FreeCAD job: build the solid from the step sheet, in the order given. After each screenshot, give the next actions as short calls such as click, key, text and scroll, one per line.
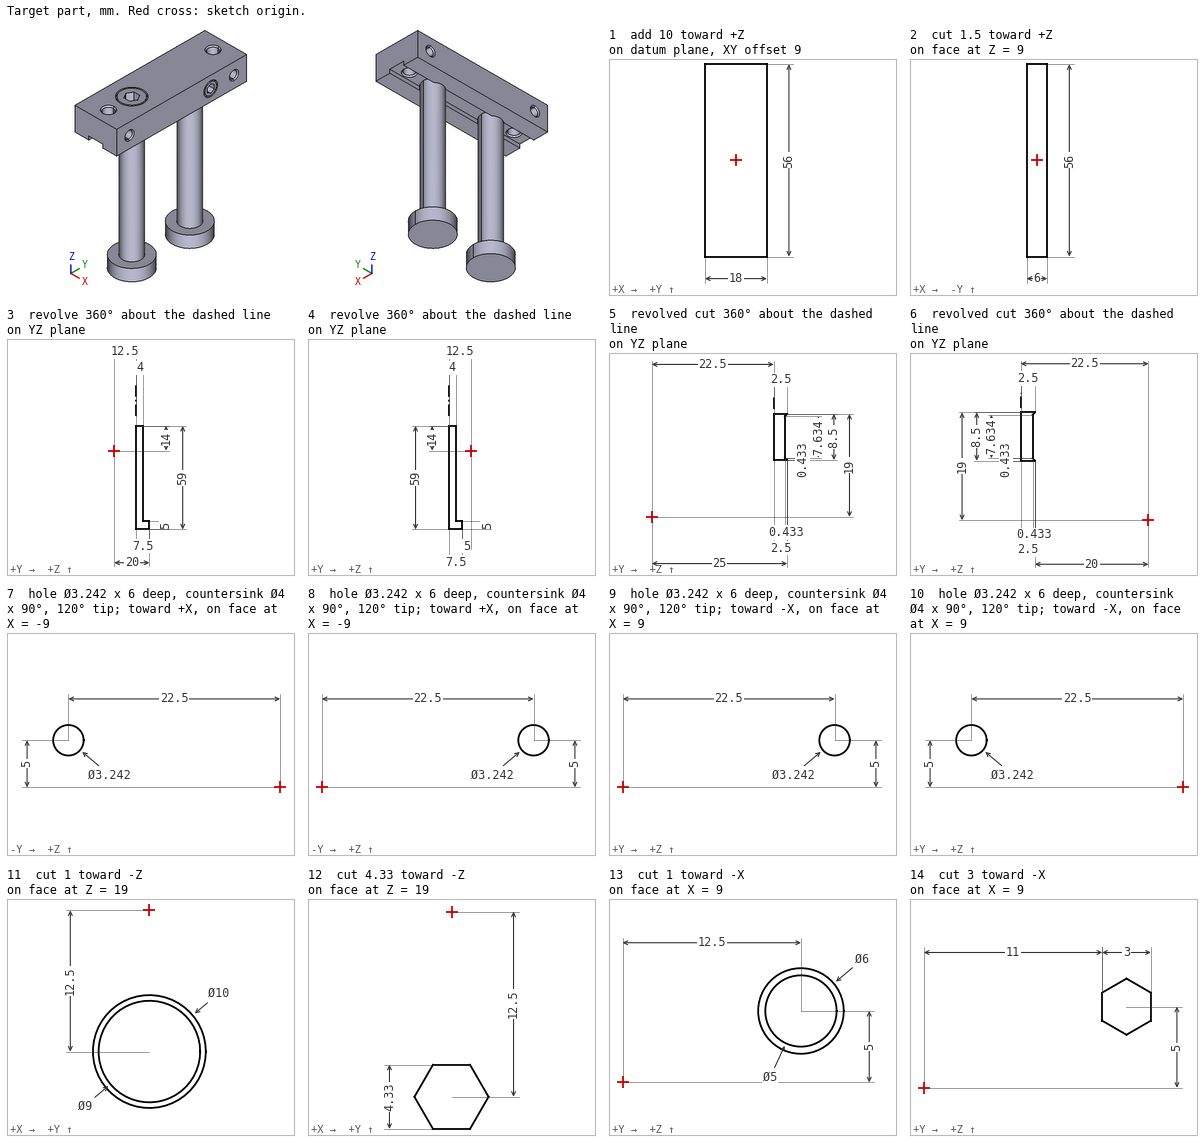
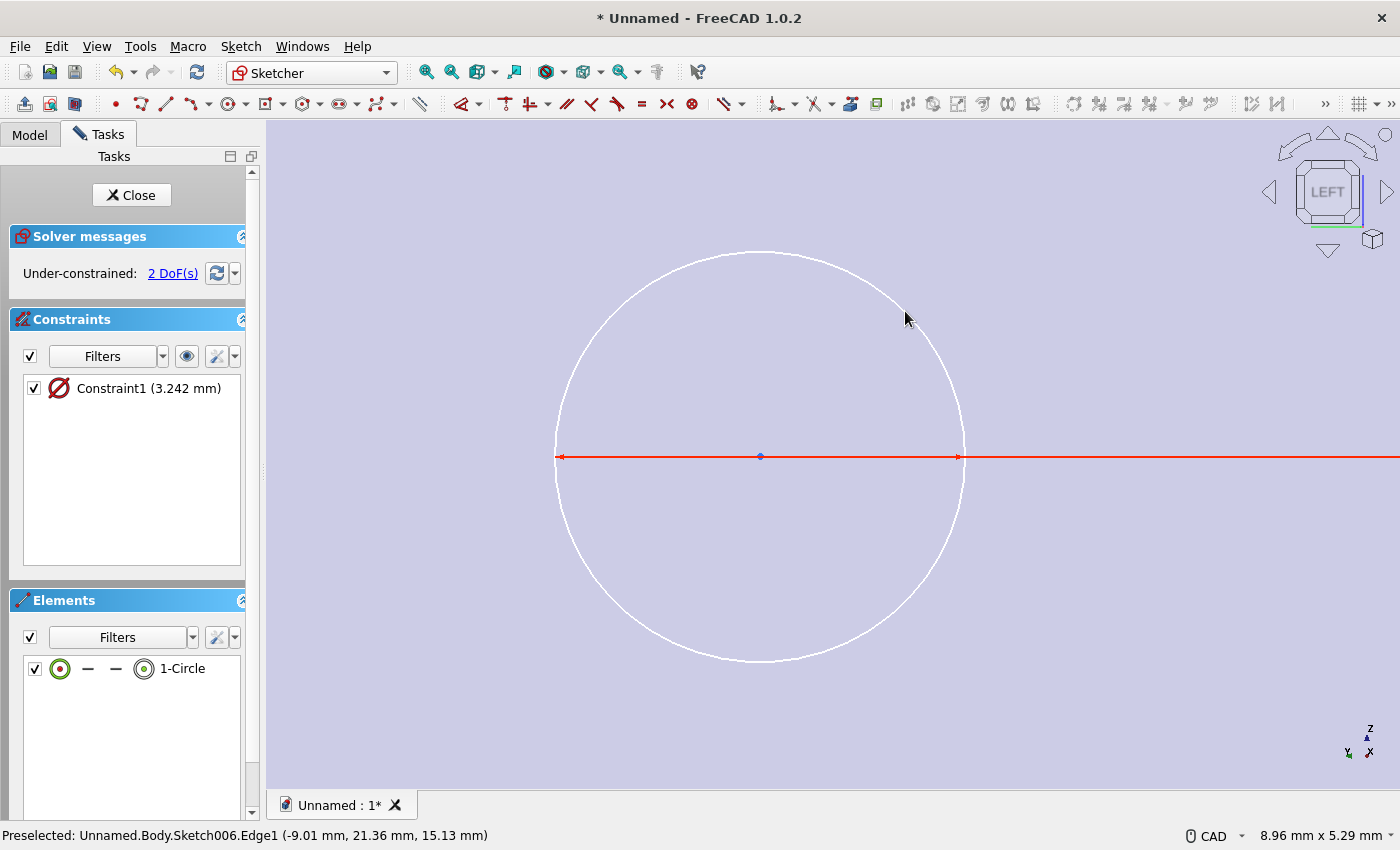
click(460, 104)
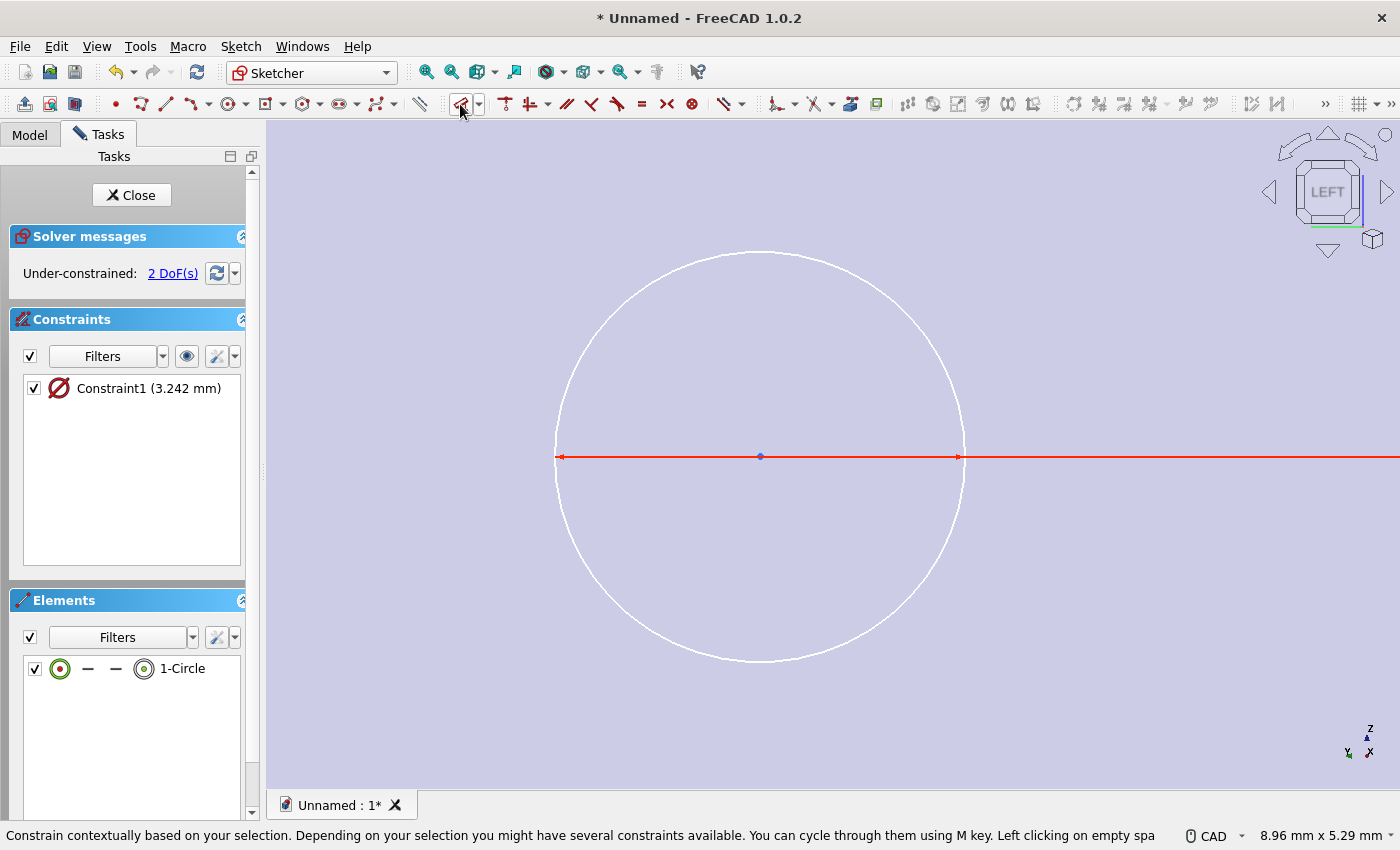
click(760, 457)
click(726, 609)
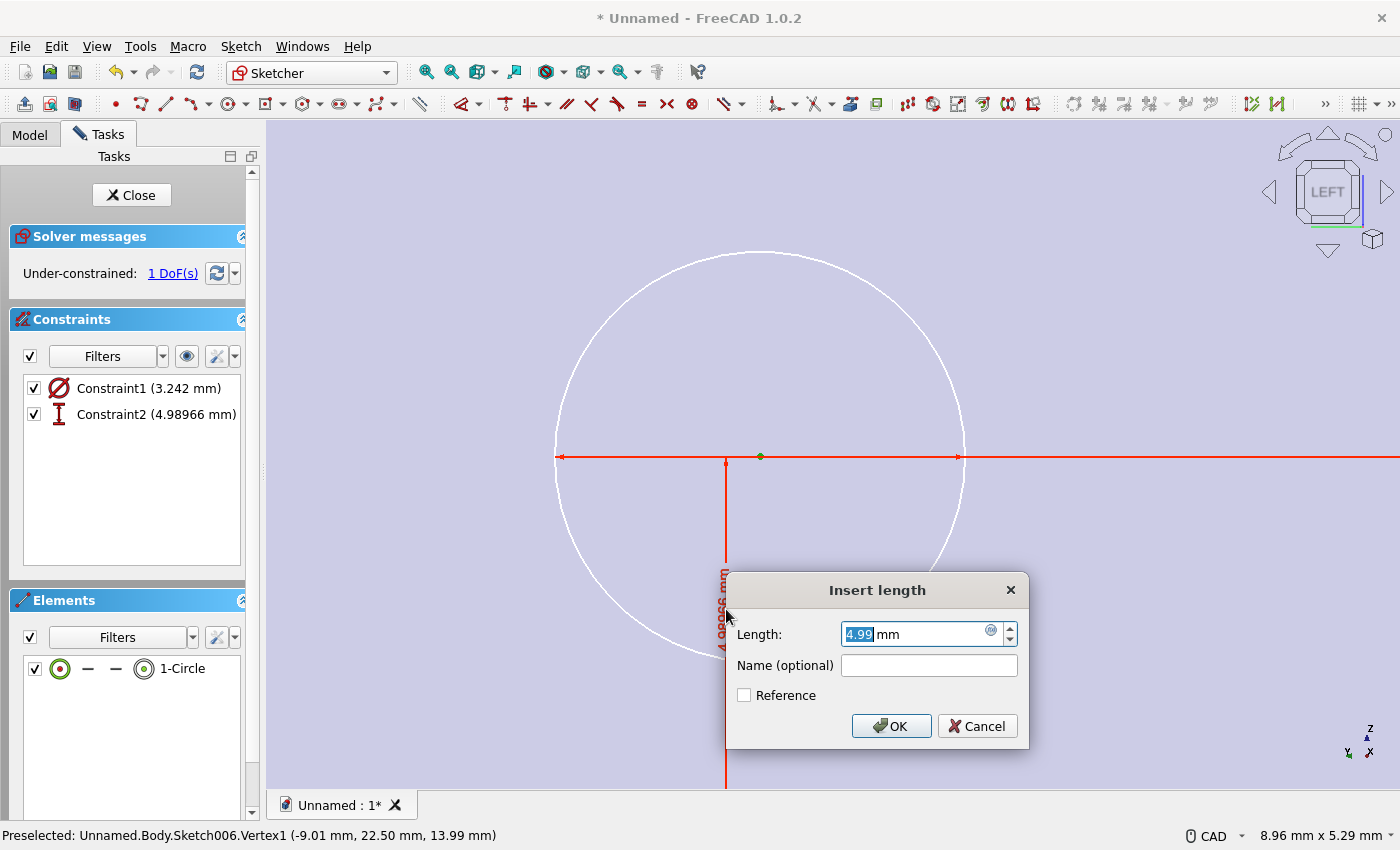
text(5)
key(Return)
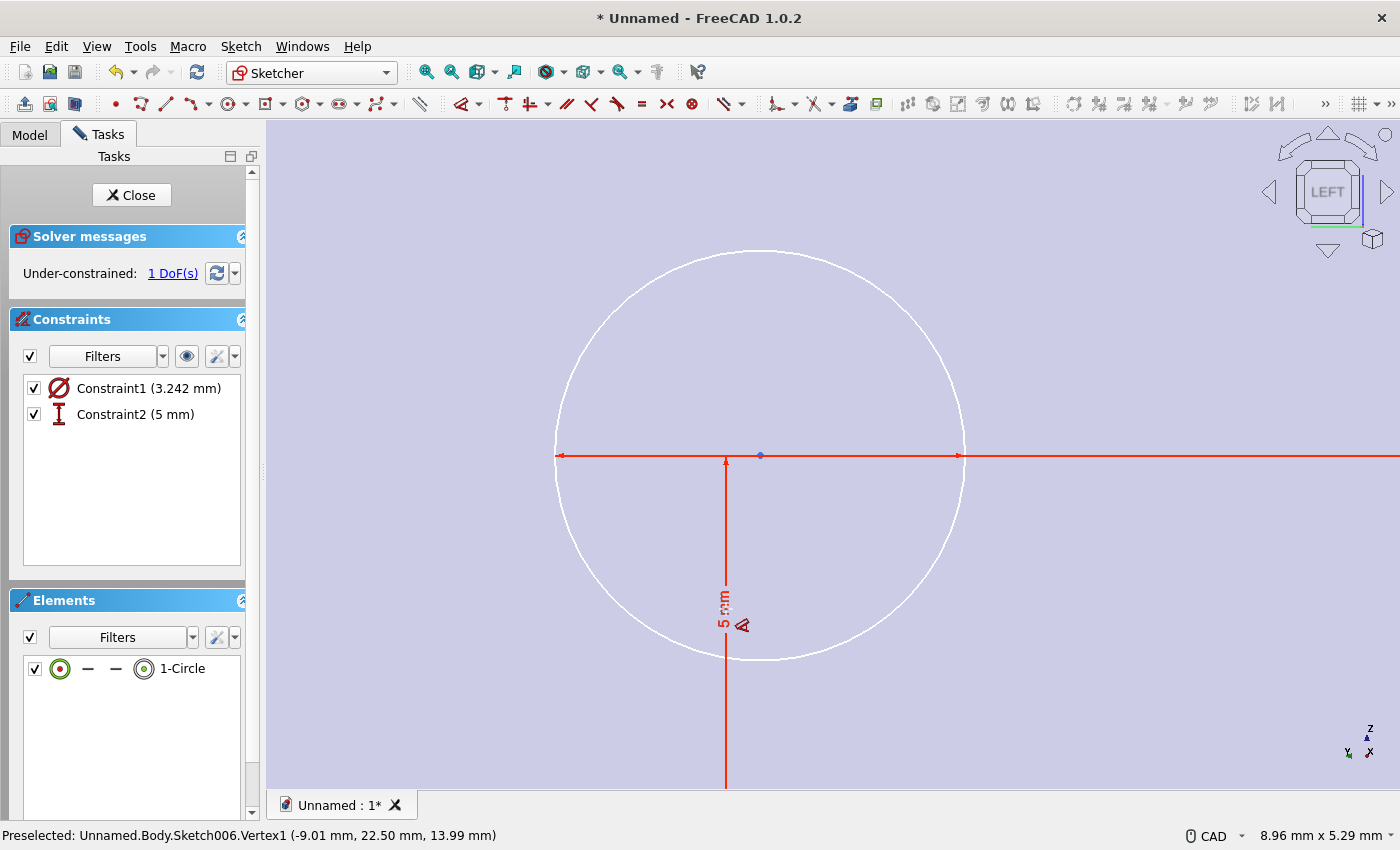
click(760, 456)
click(998, 422)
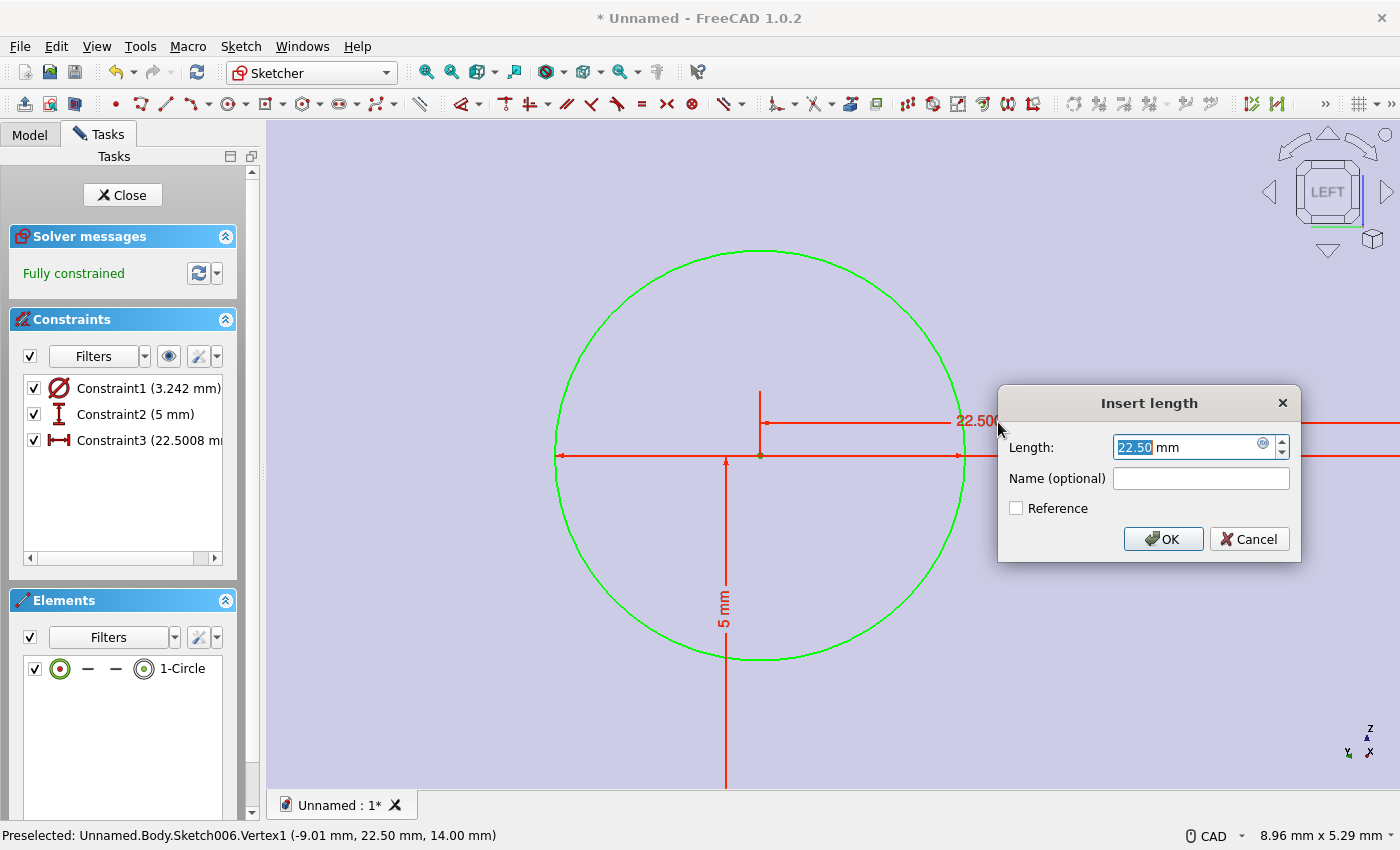
text(22.5)
key(Return)
key(Escape)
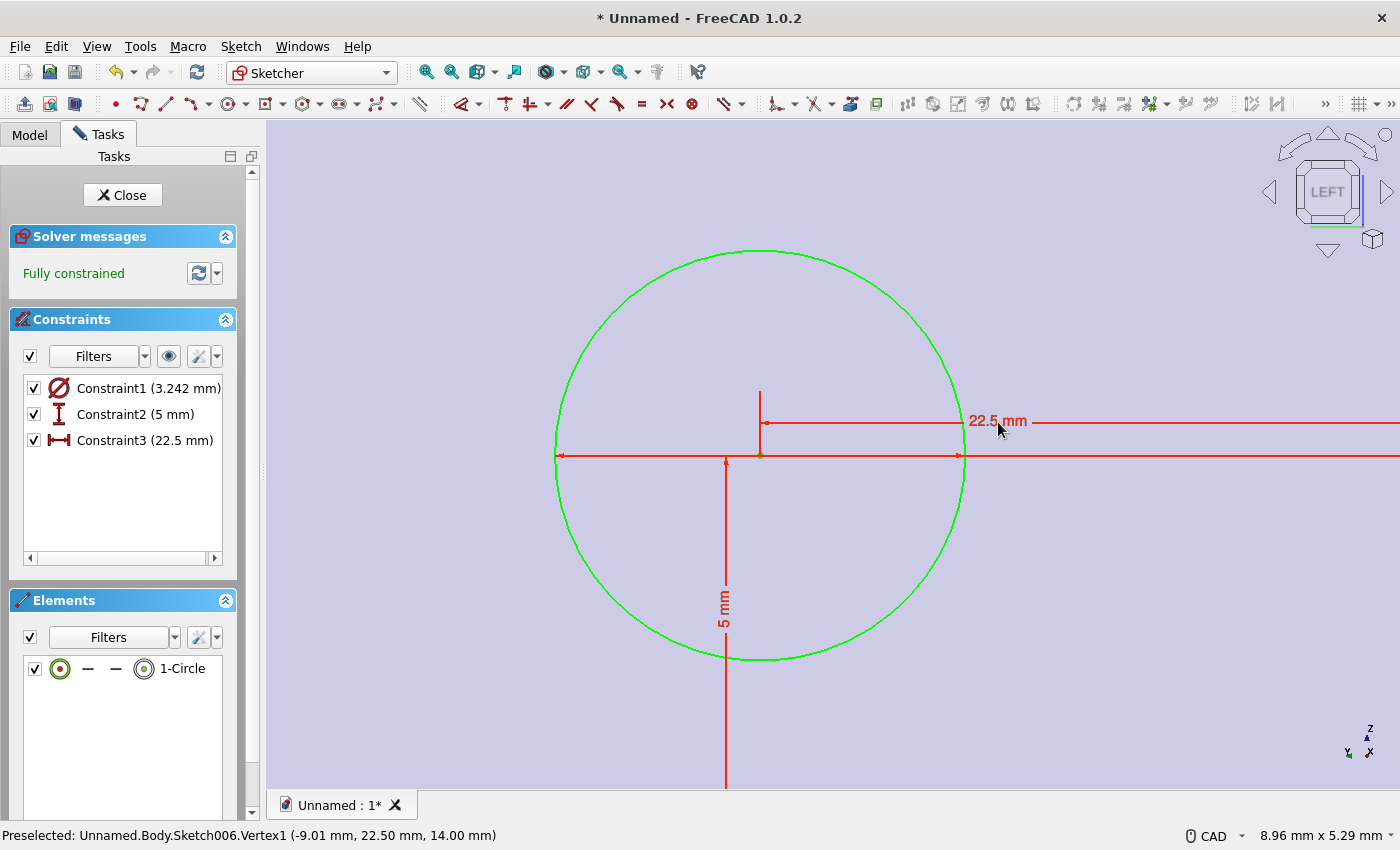
click(123, 195)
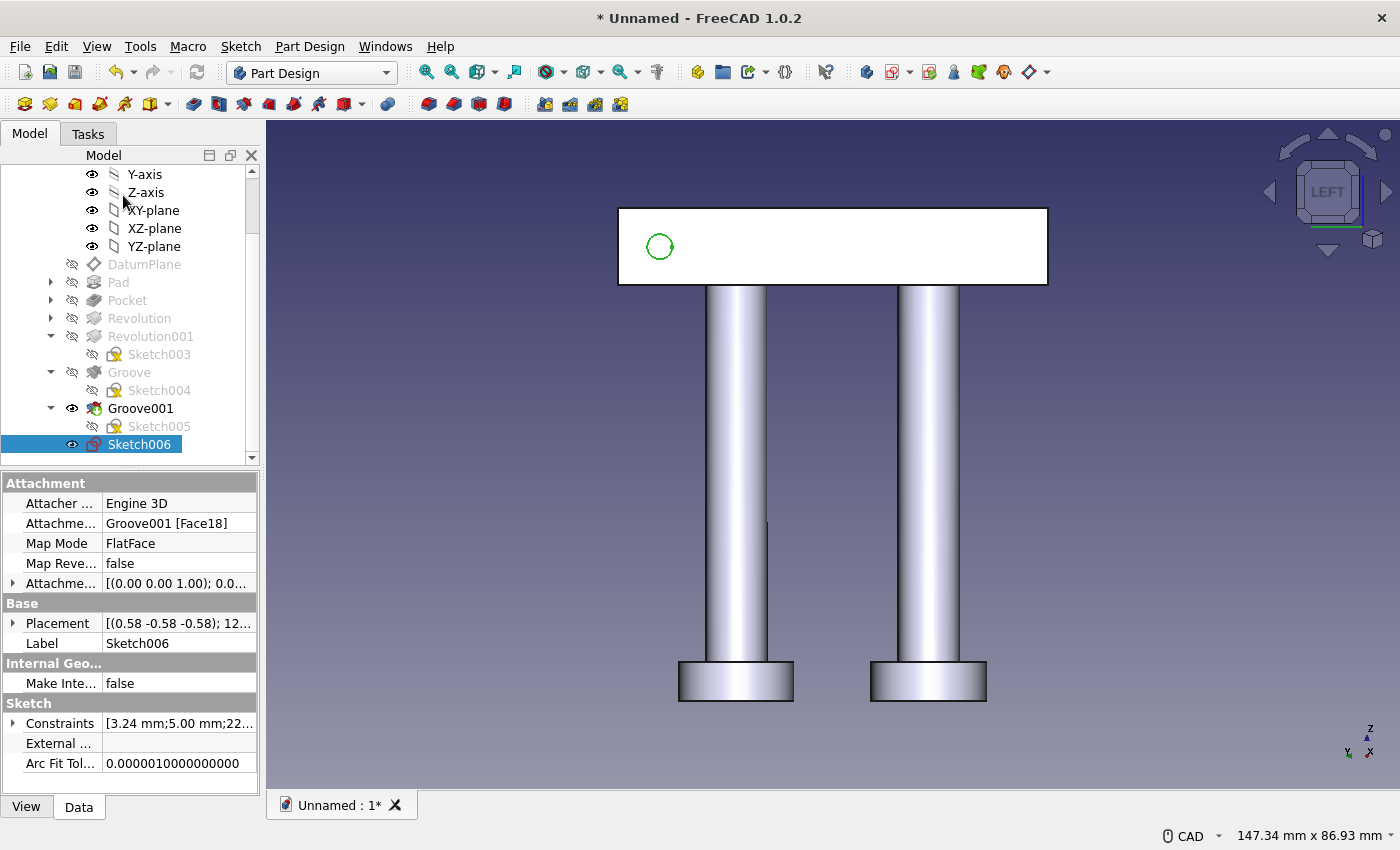
click(219, 104)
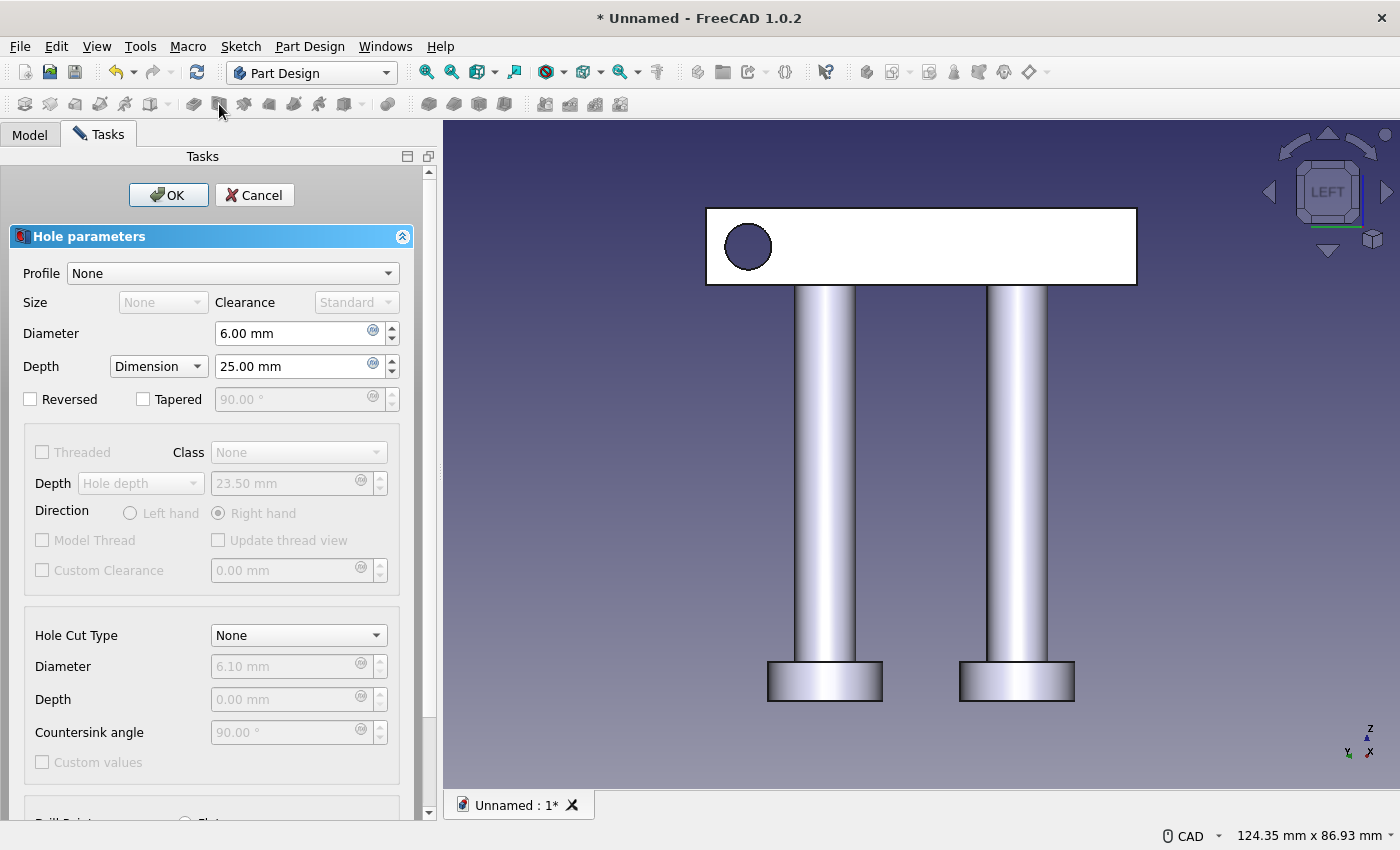
triple_click(300, 334)